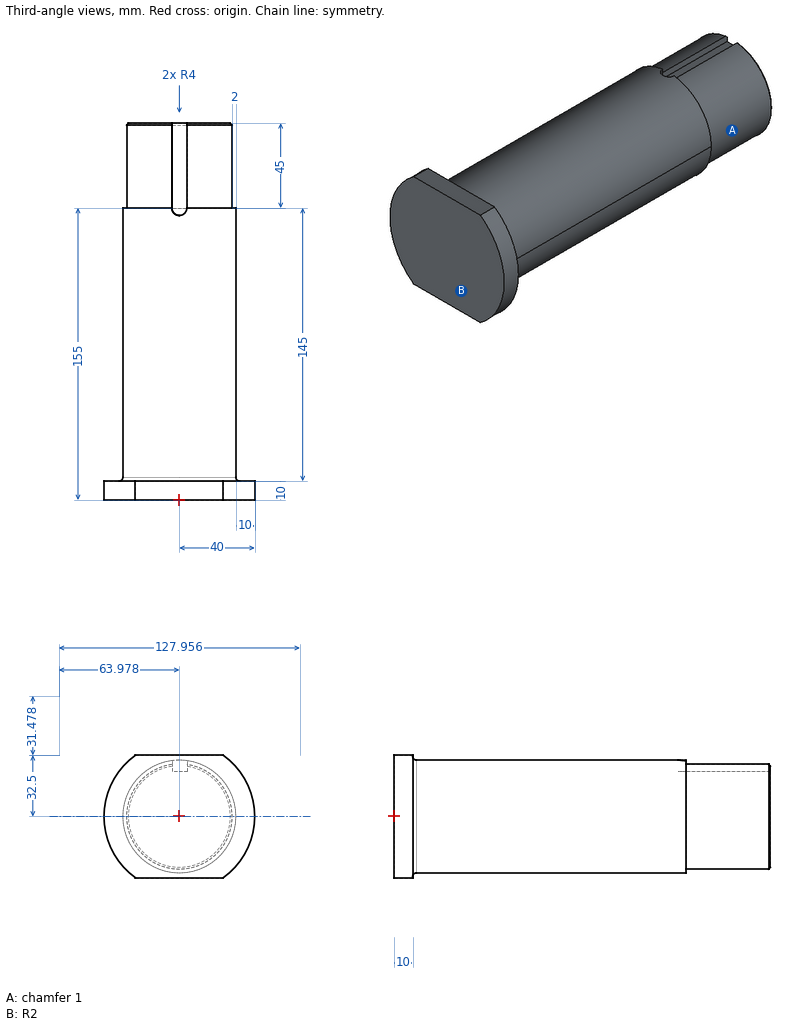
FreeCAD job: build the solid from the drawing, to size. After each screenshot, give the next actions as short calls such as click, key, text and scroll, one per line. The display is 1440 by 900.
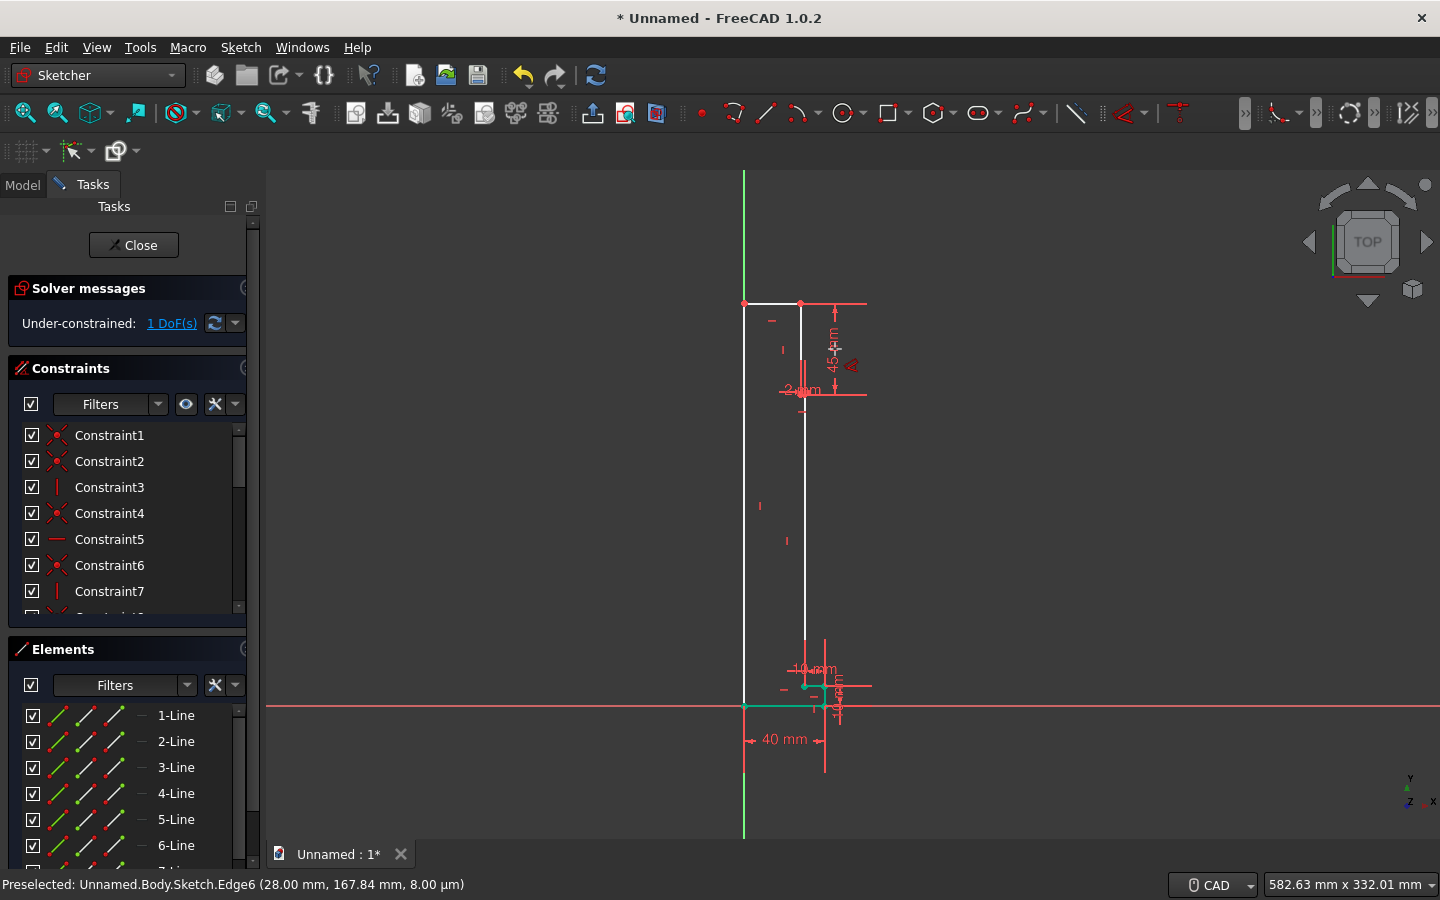
click(805, 599)
click(839, 540)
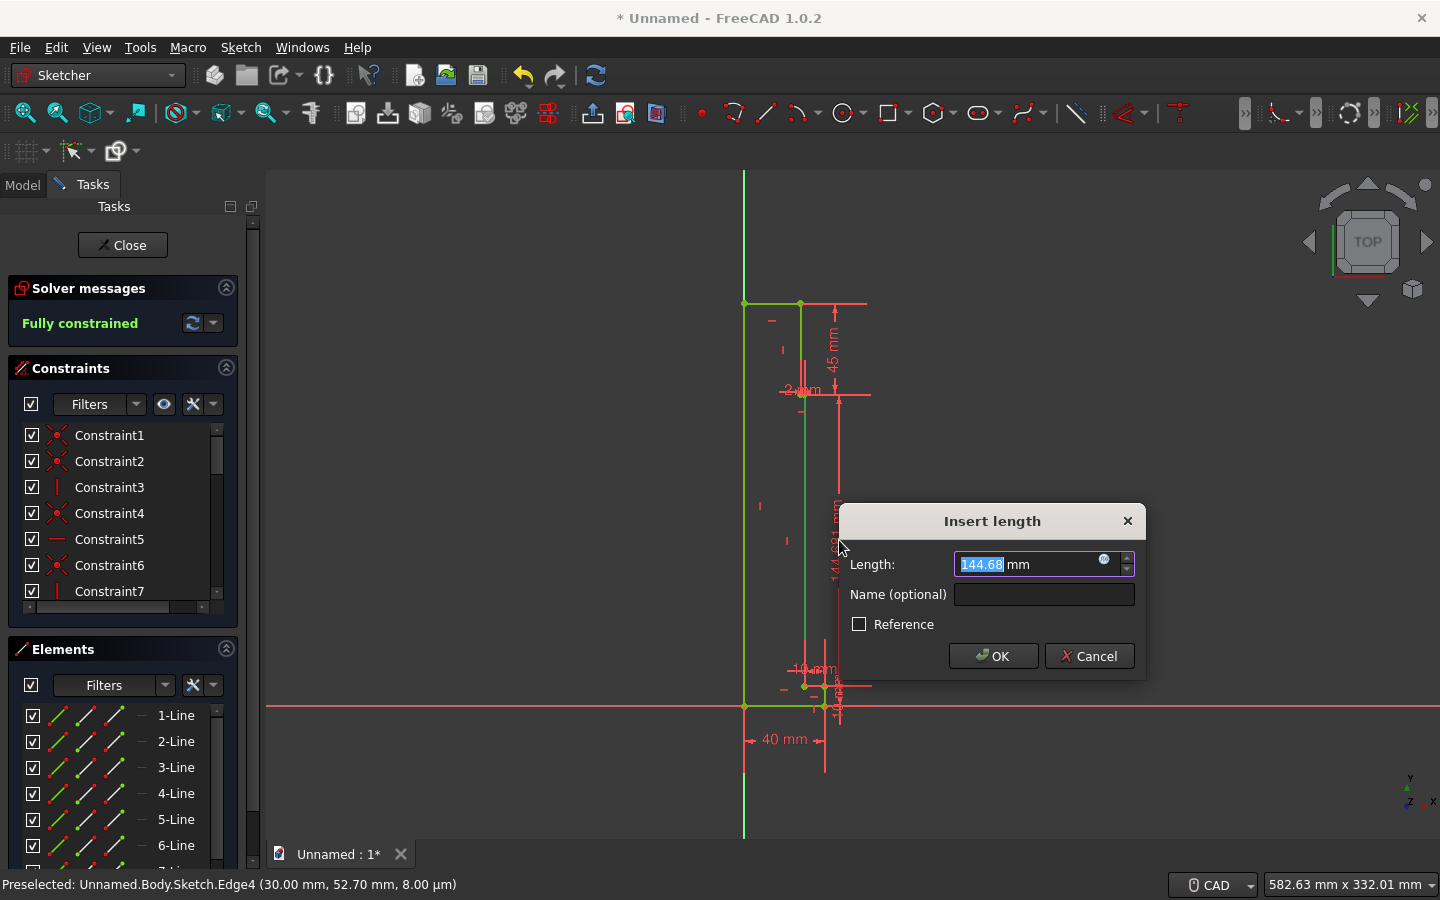
text(145)
key(Return)
key(Escape)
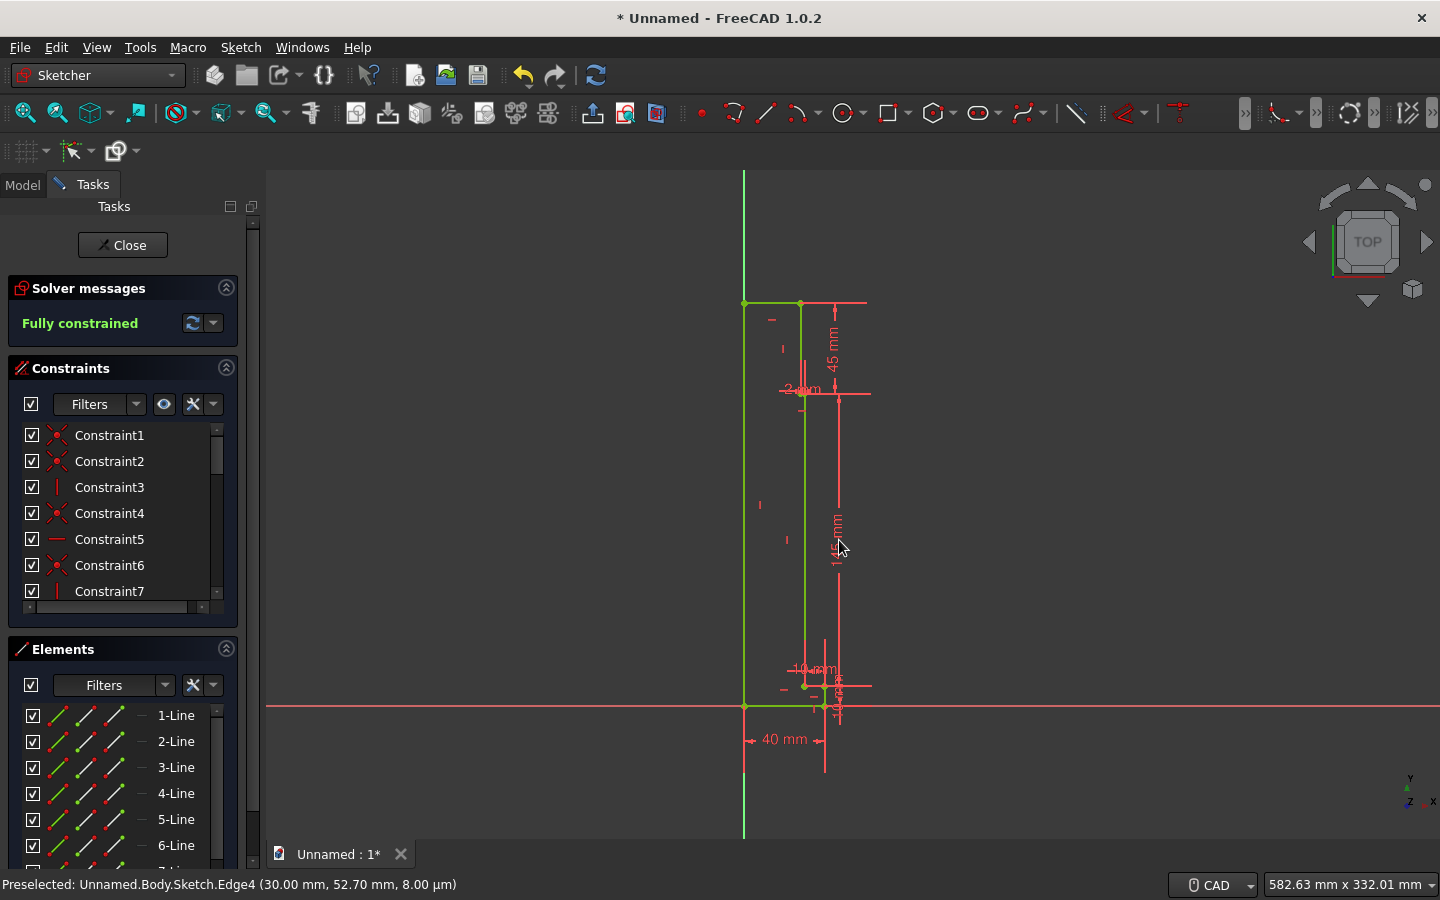
click(123, 245)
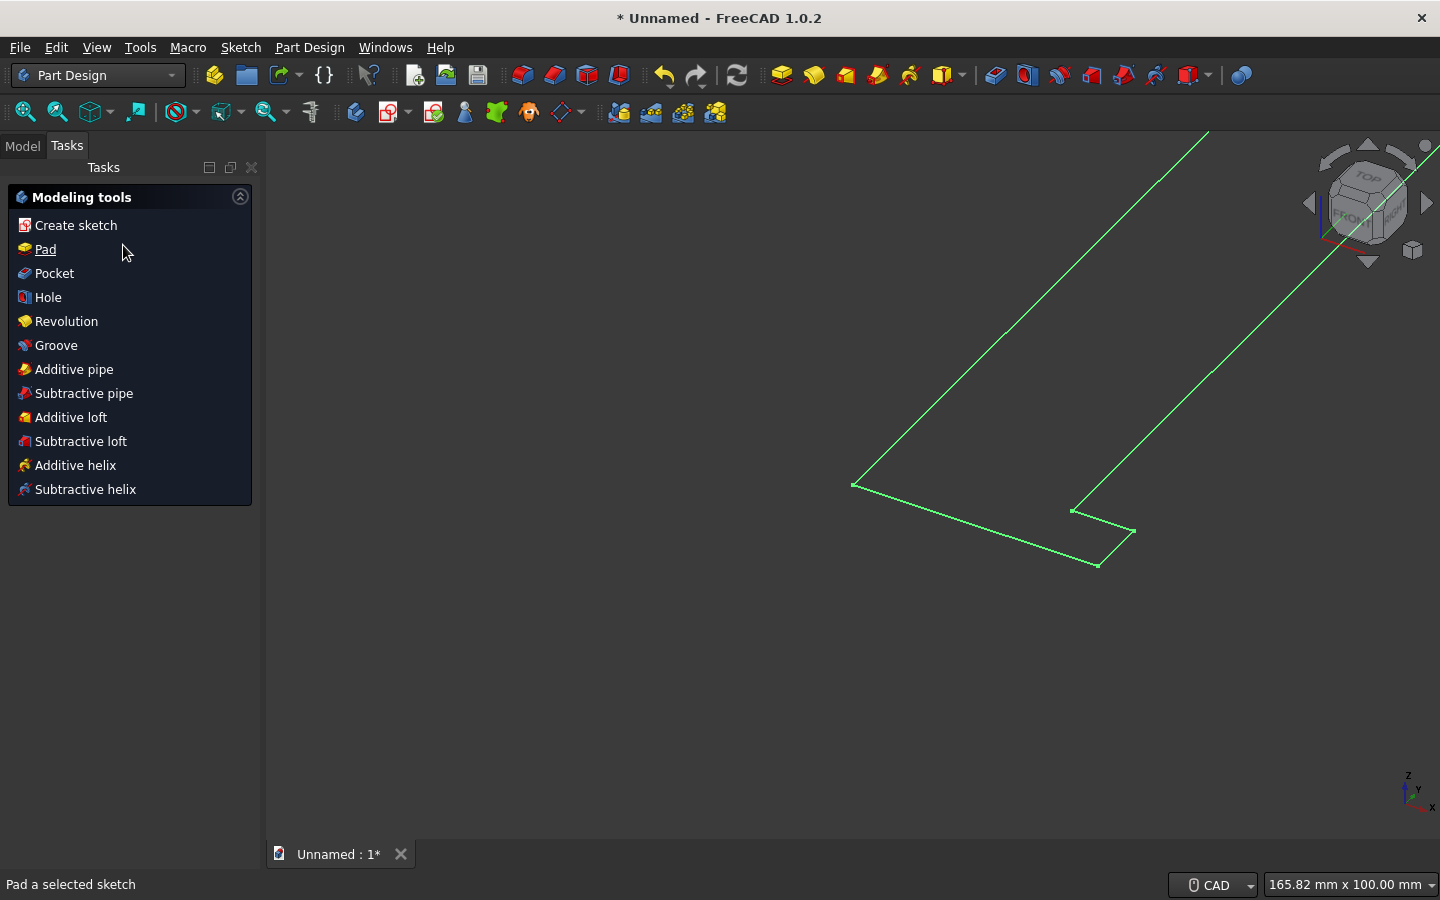
click(814, 76)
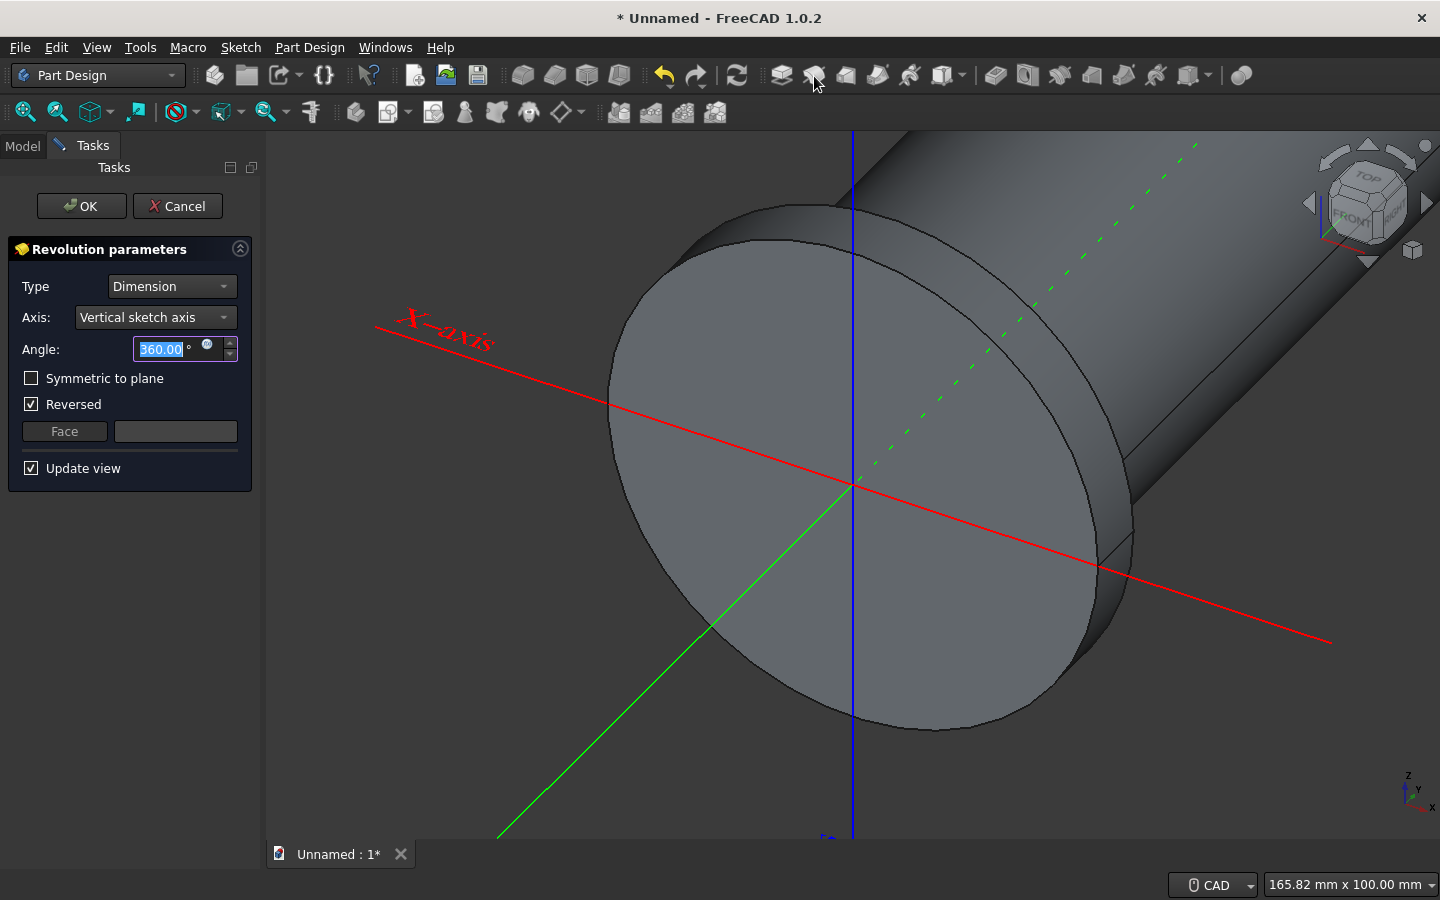
click(82, 206)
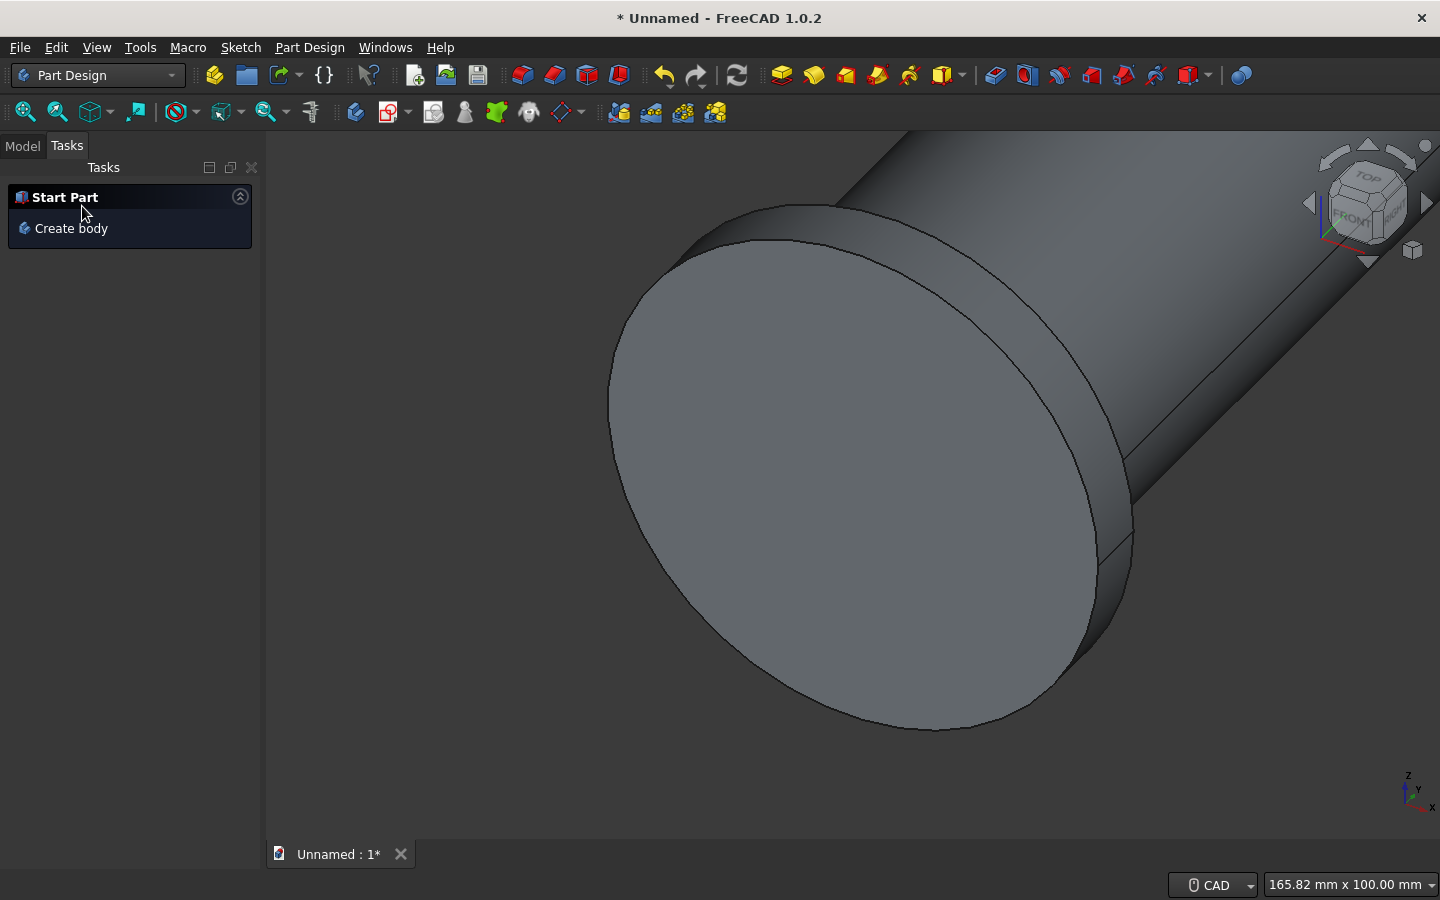
click(26, 112)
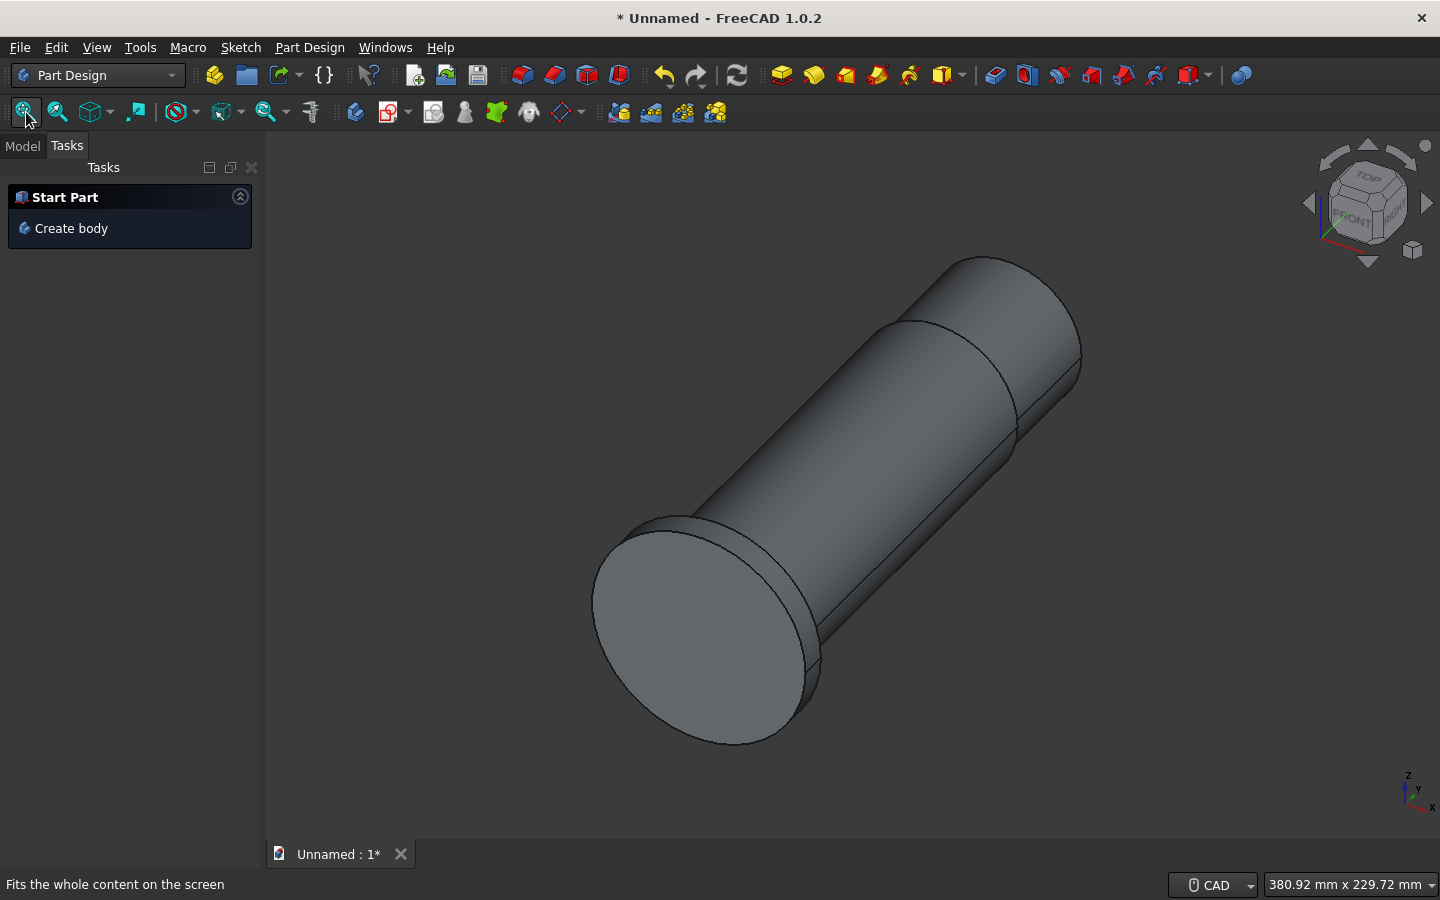
click(699, 637)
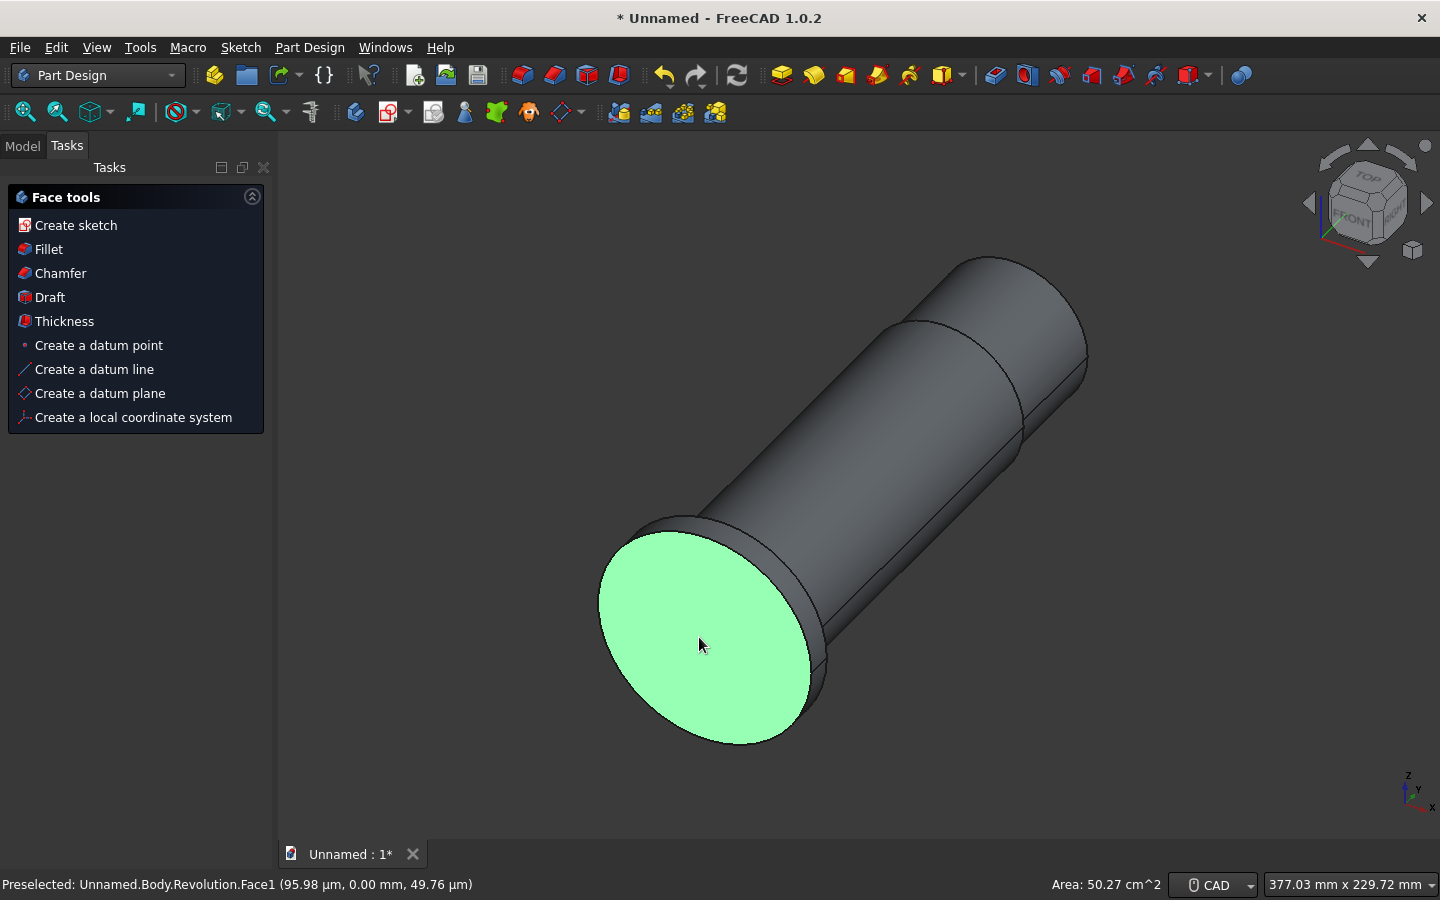
click(388, 112)